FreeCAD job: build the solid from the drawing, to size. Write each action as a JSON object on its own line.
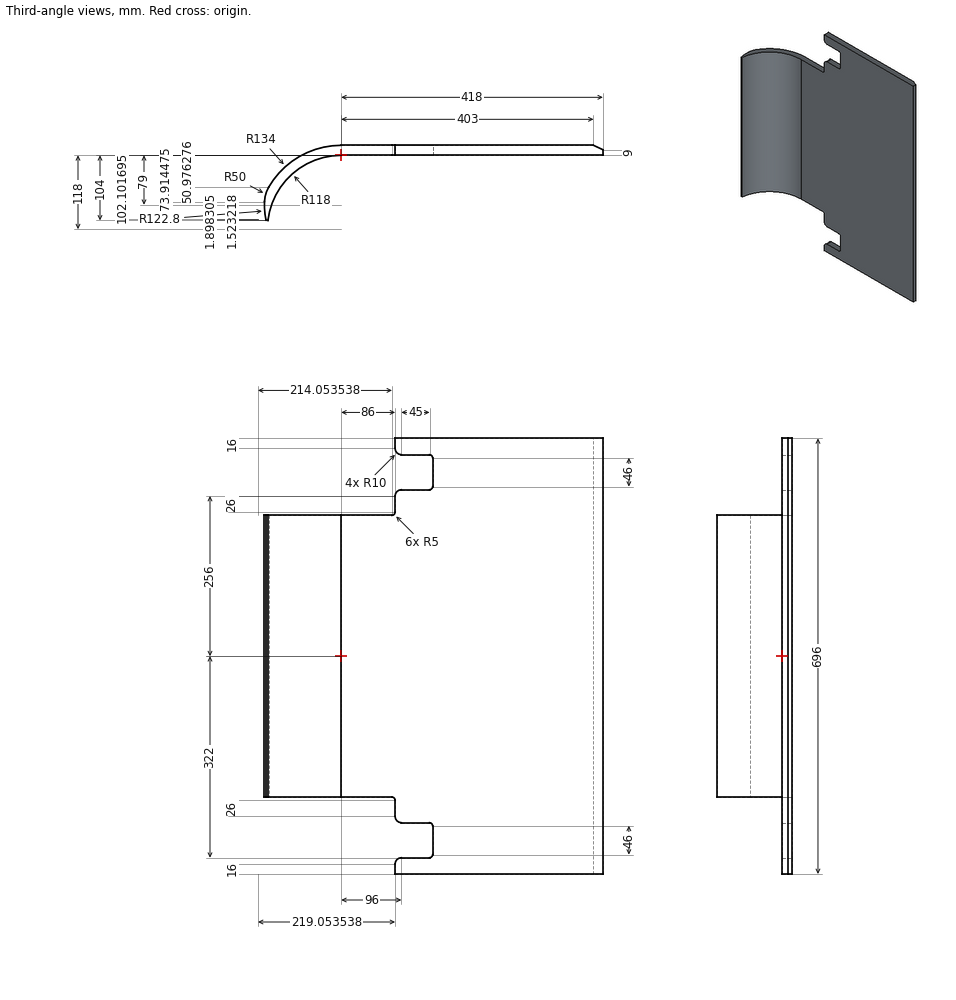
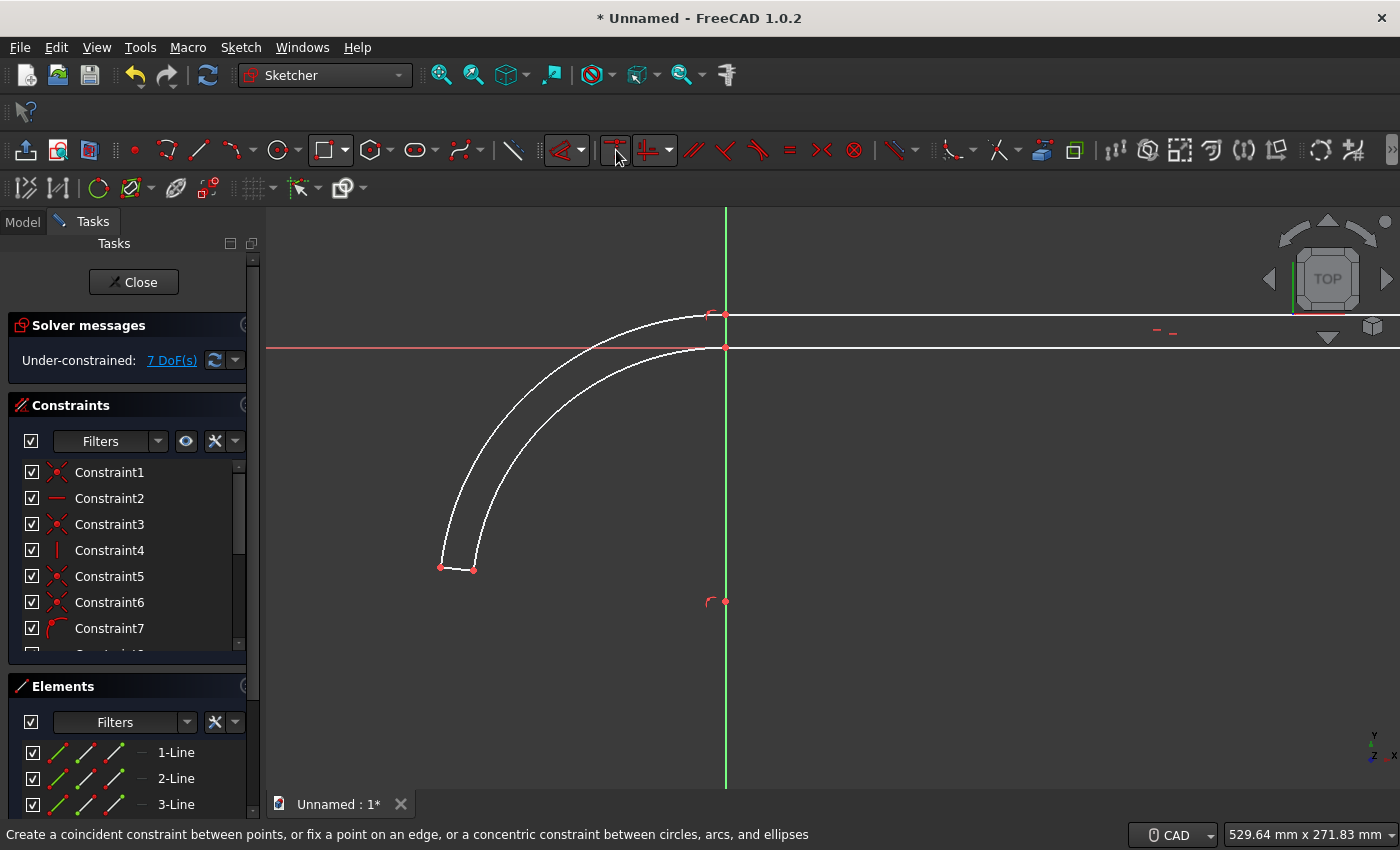
{"action": "left_click", "coordinate": [560, 150]}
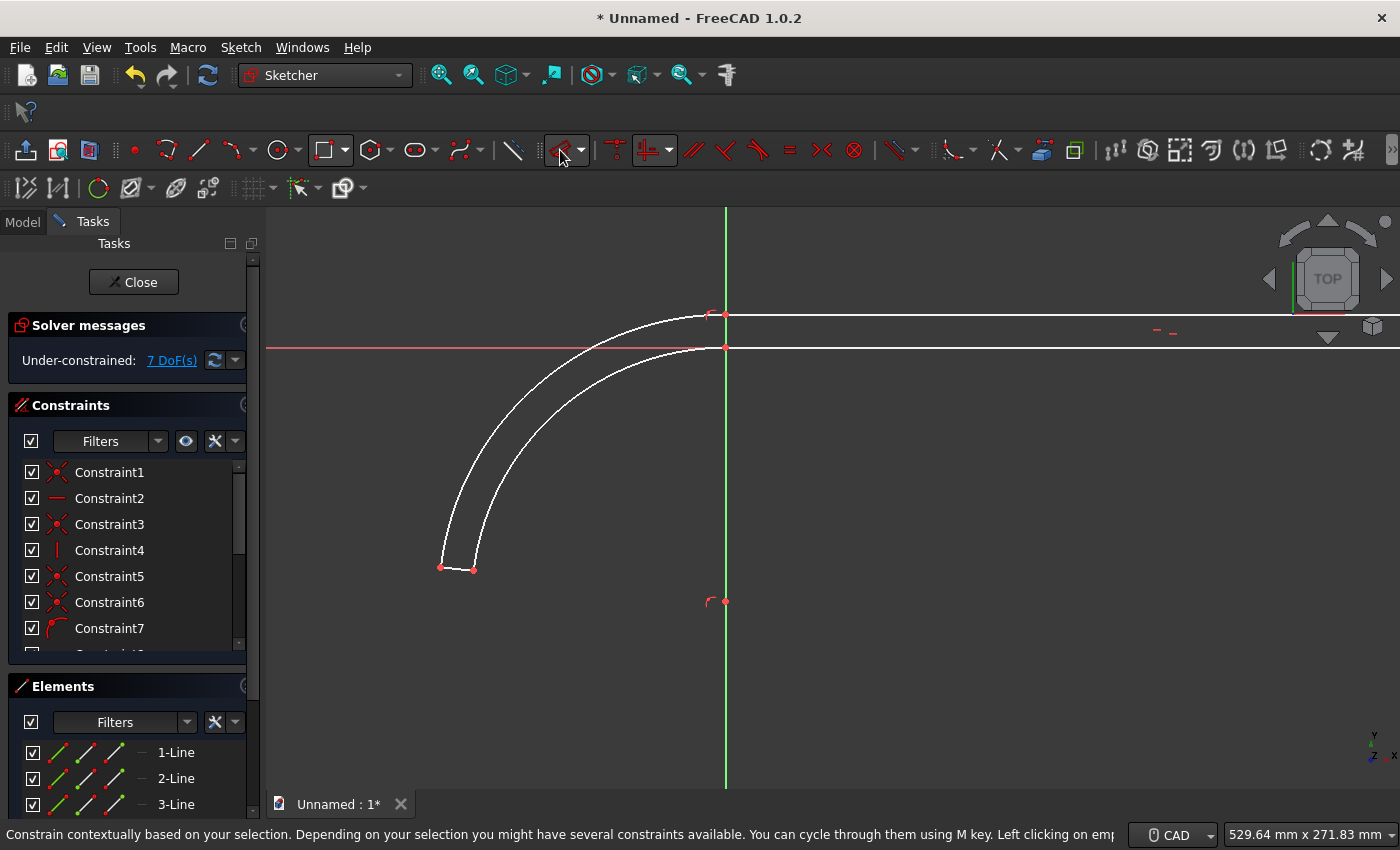
{"action": "left_click", "coordinate": [482, 450]}
{"action": "left_click", "coordinate": [455, 433]}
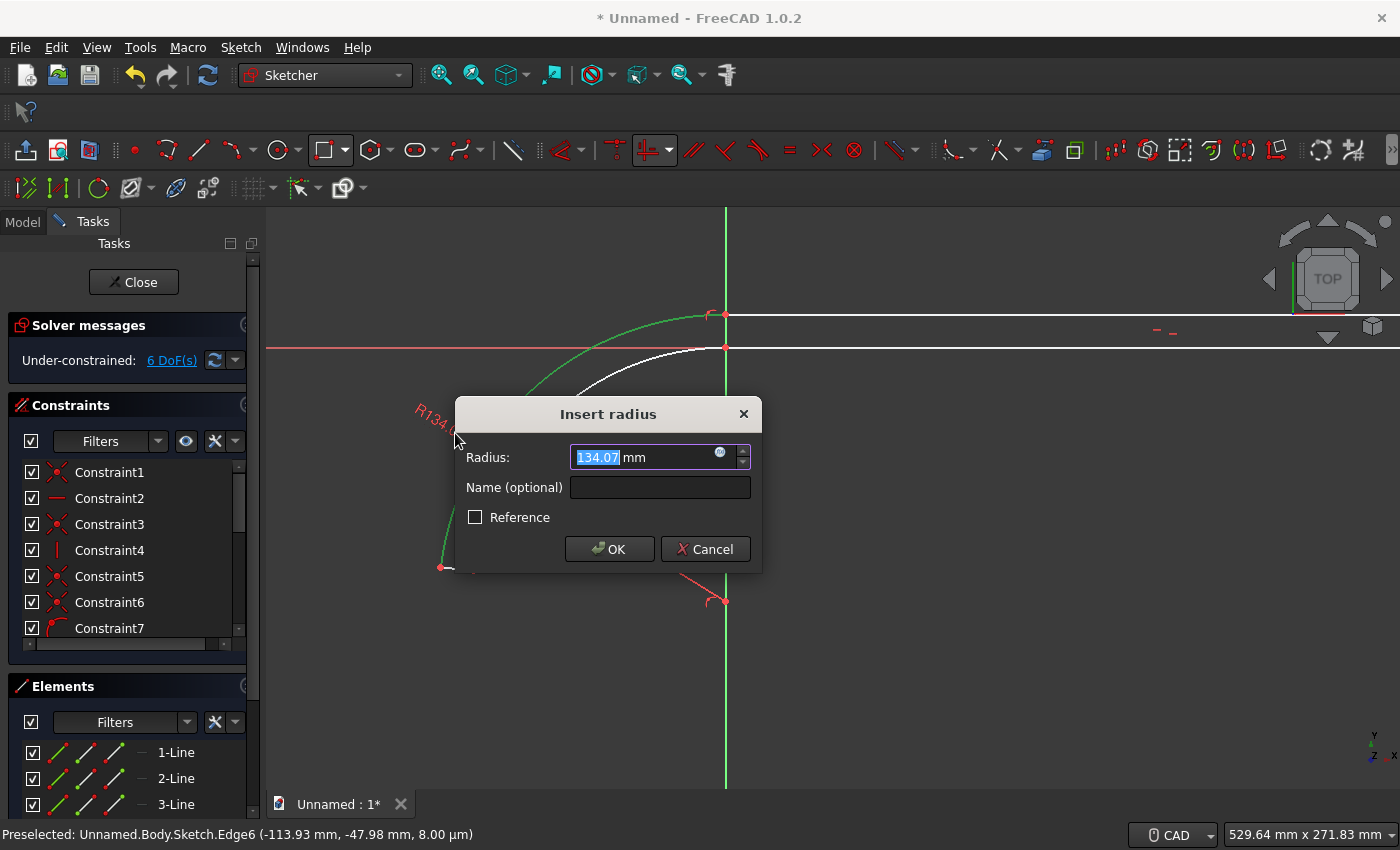
{"action": "type", "text": "134"}
{"action": "key", "text": "Return"}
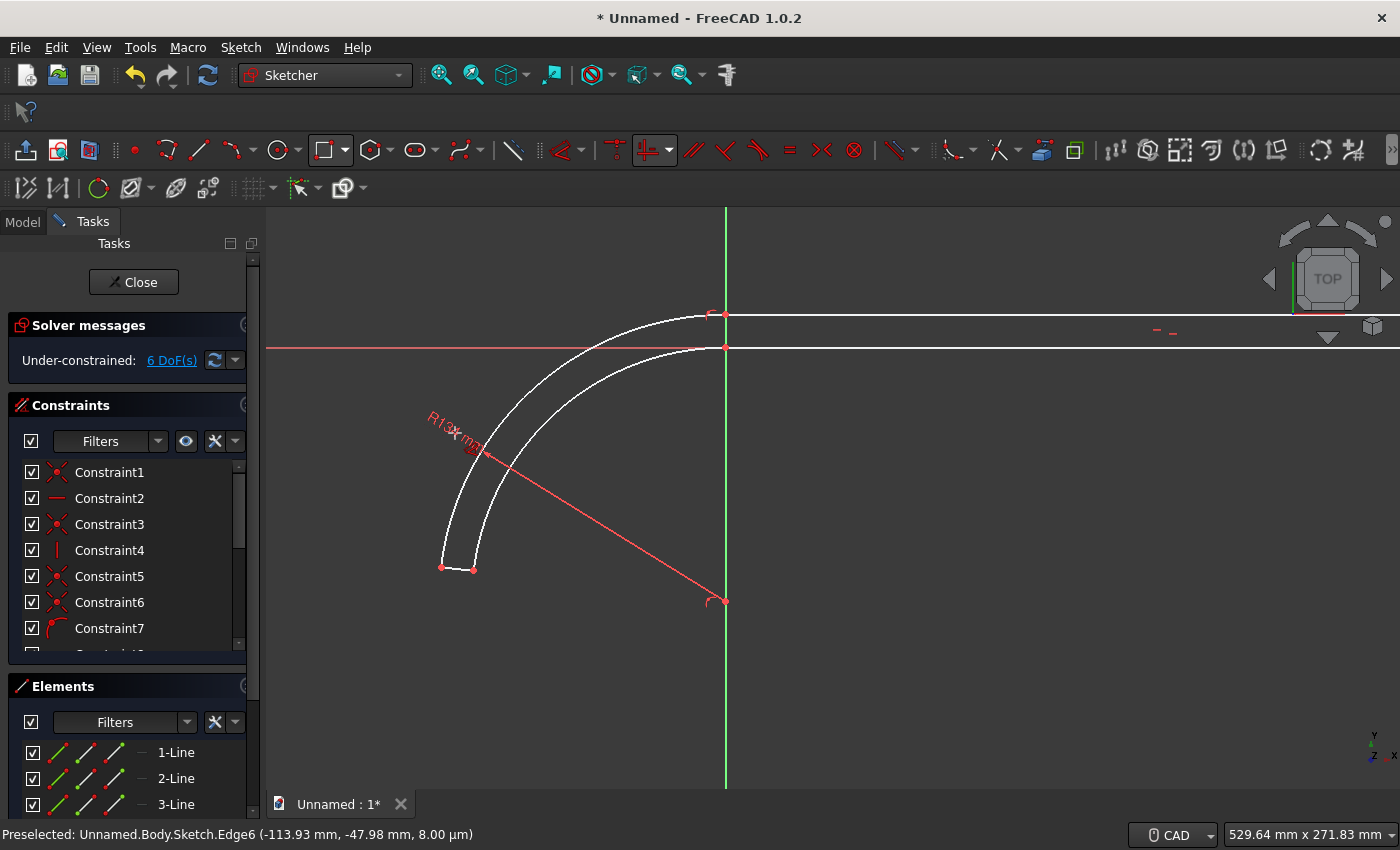
{"action": "left_click", "coordinate": [619, 371]}
{"action": "left_click", "coordinate": [985, 481]}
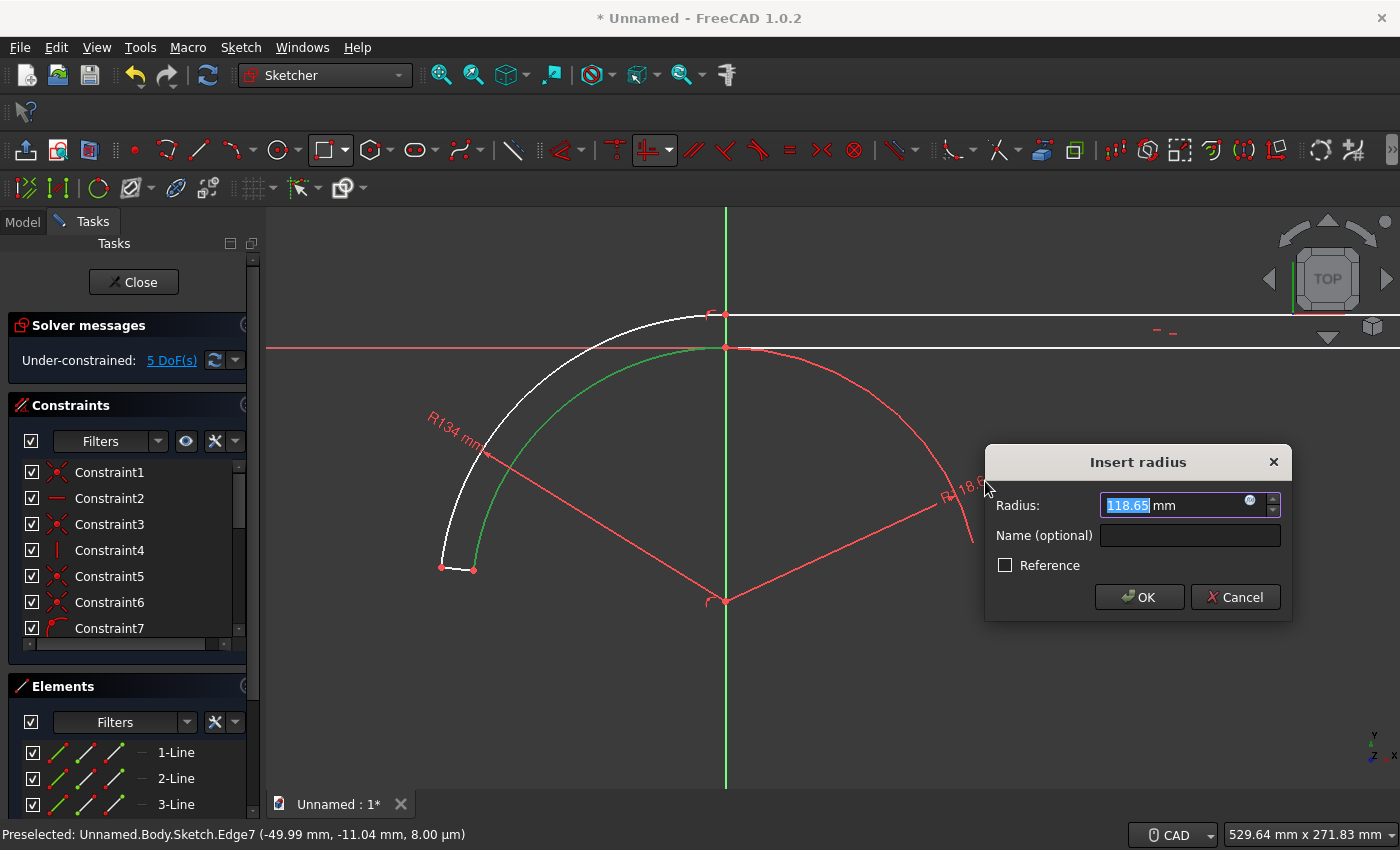
{"action": "type", "text": "118"}
{"action": "key", "text": "Return"}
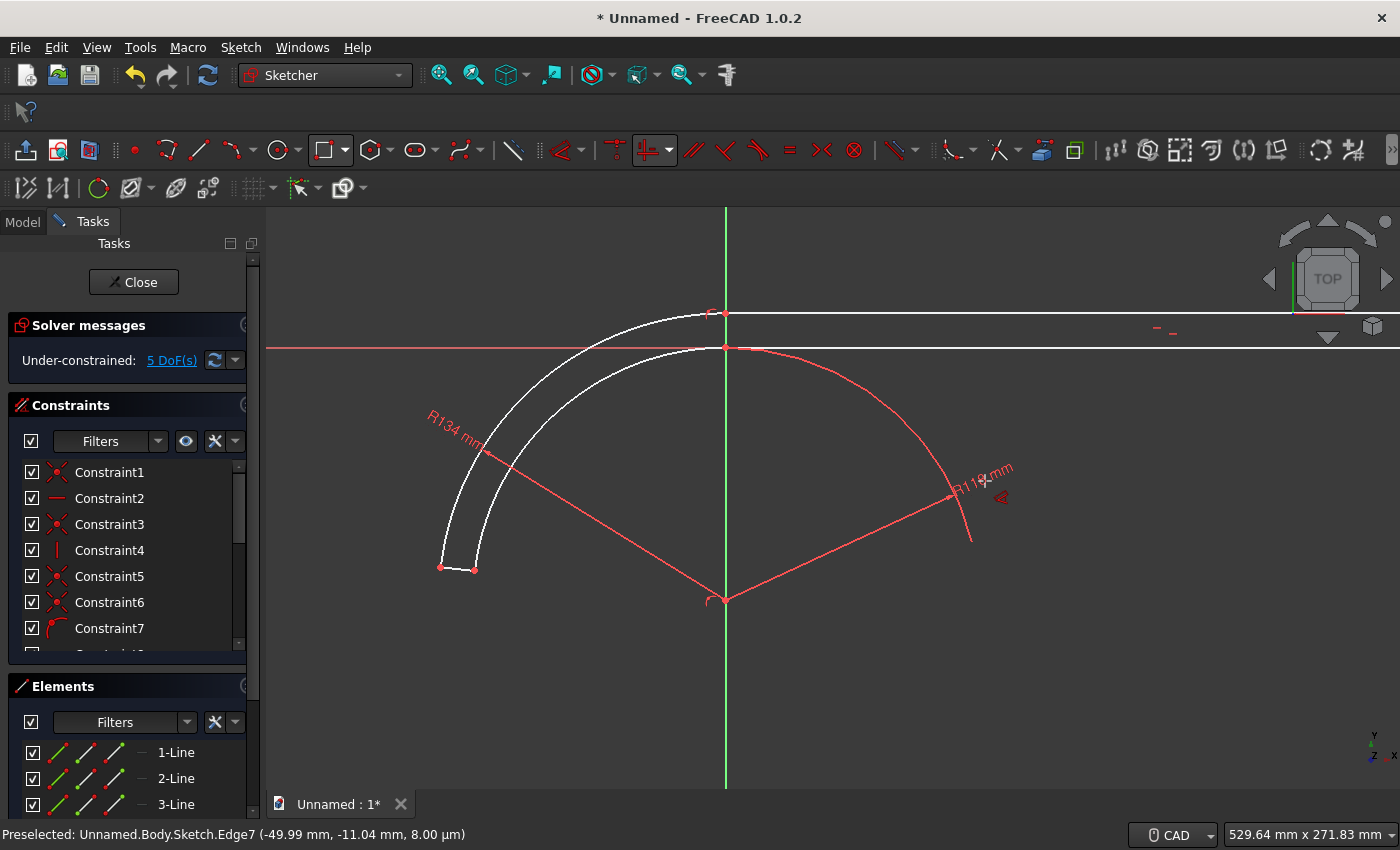
{"action": "scroll", "coordinate": [440, 566], "scroll_direction": "down", "scroll_amount": 3}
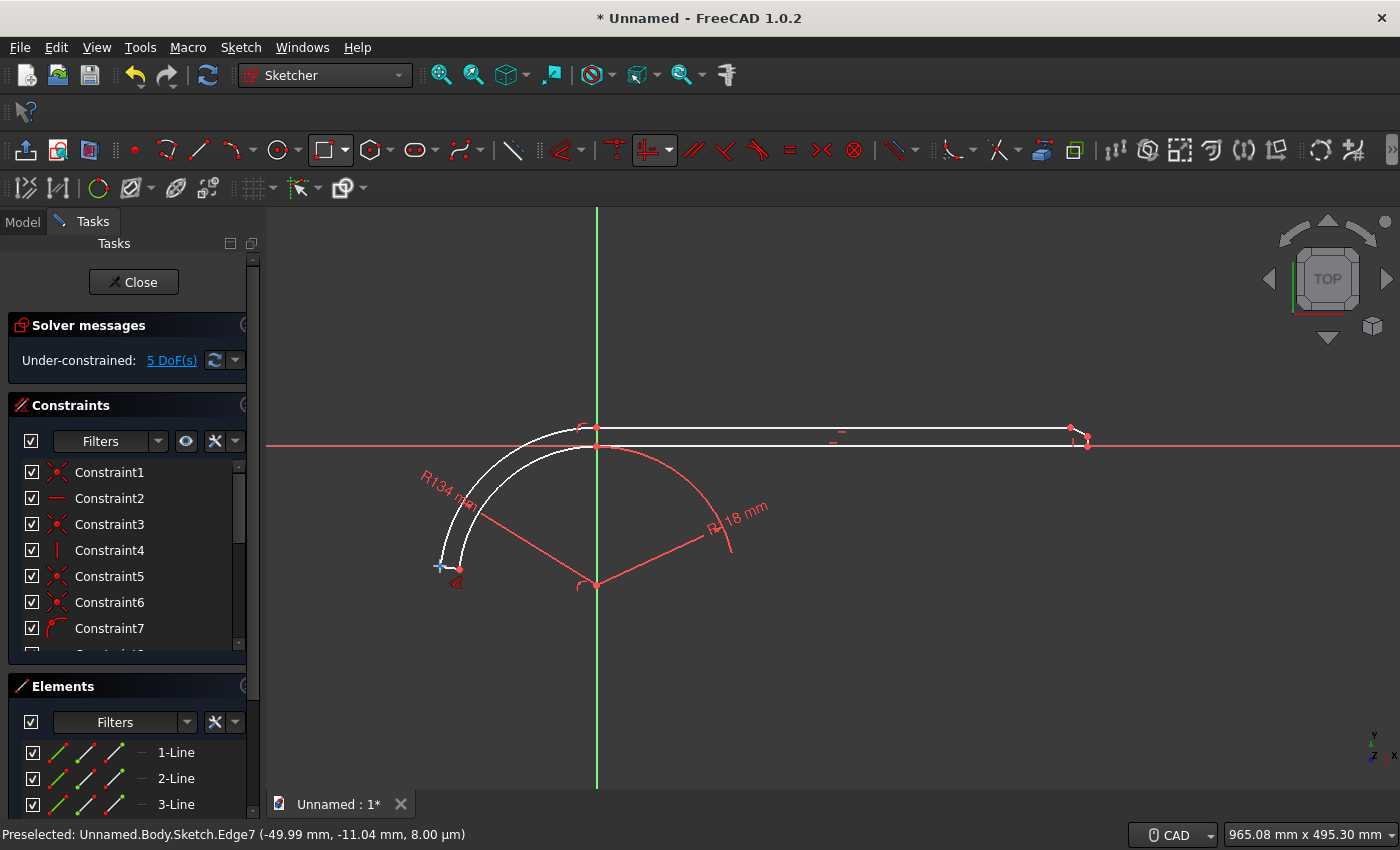
{"action": "scroll", "coordinate": [1088, 441], "scroll_direction": "up", "scroll_amount": 7}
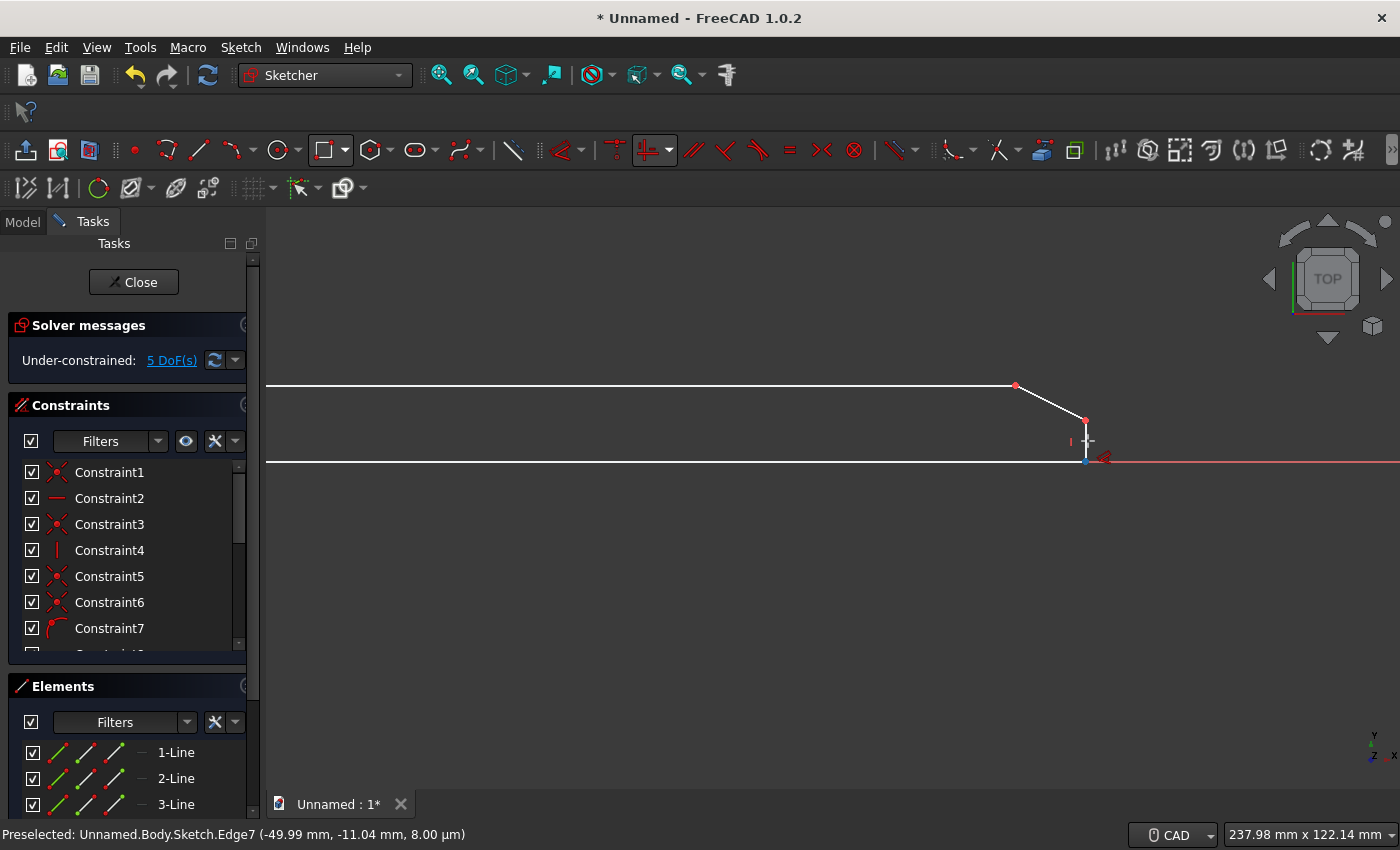
{"action": "left_click", "coordinate": [1086, 441]}
{"action": "left_click", "coordinate": [1120, 441]}